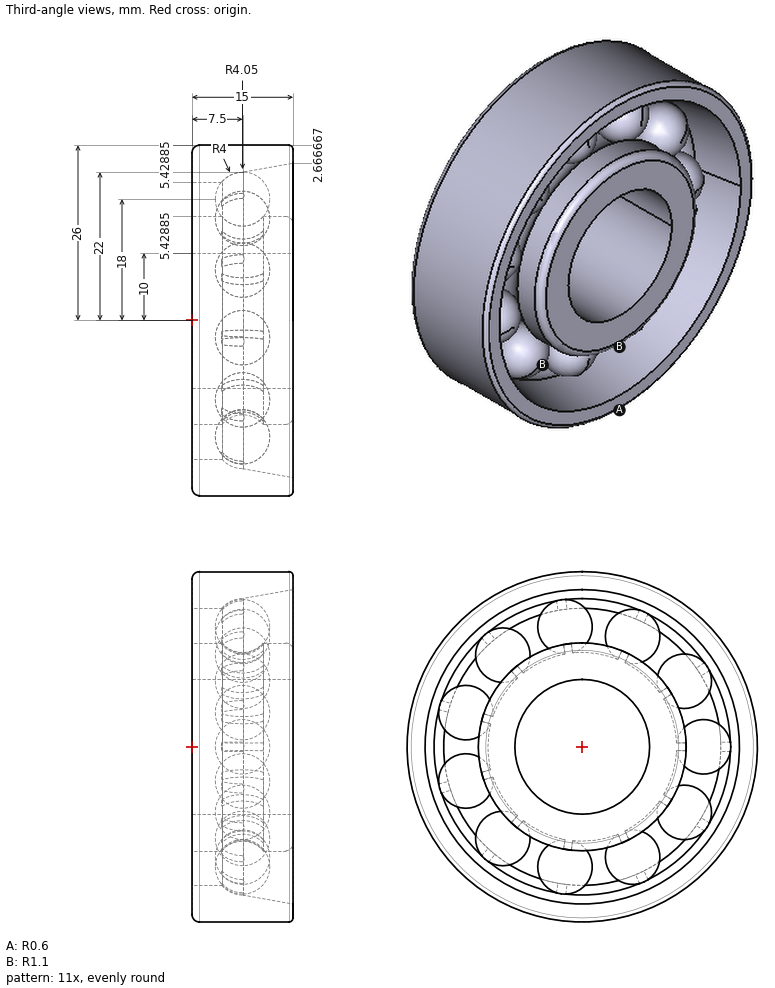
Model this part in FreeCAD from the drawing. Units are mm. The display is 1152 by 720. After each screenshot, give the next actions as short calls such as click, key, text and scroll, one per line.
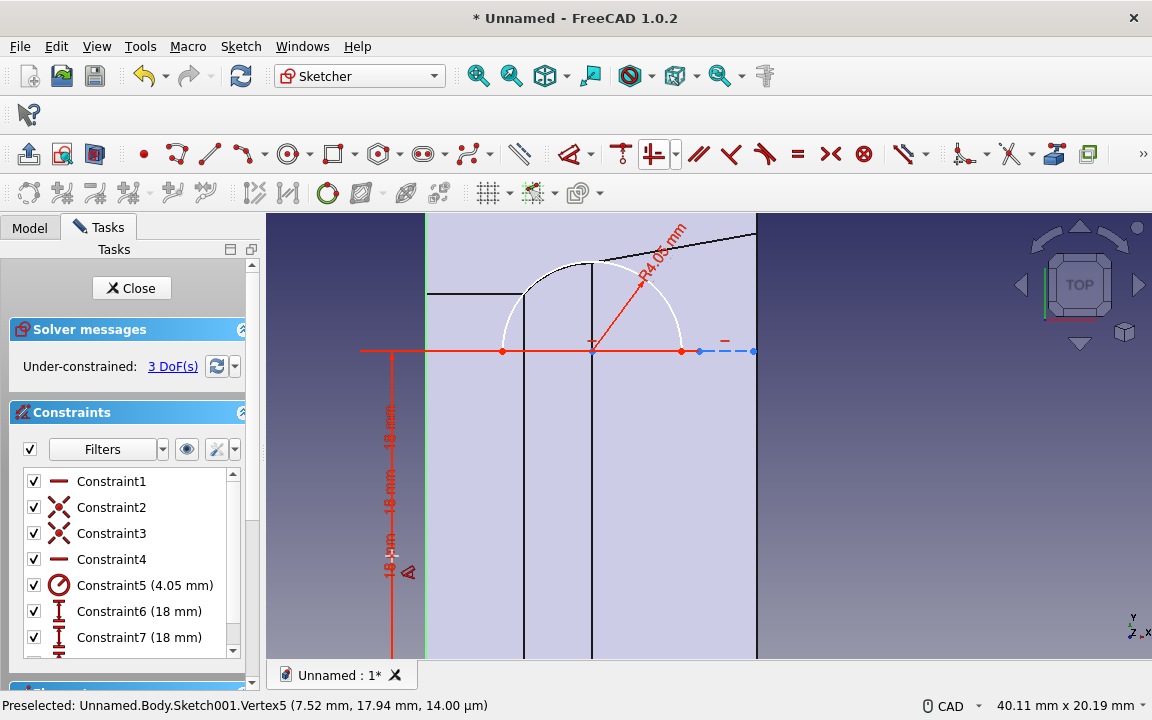
click(592, 351)
click(471, 317)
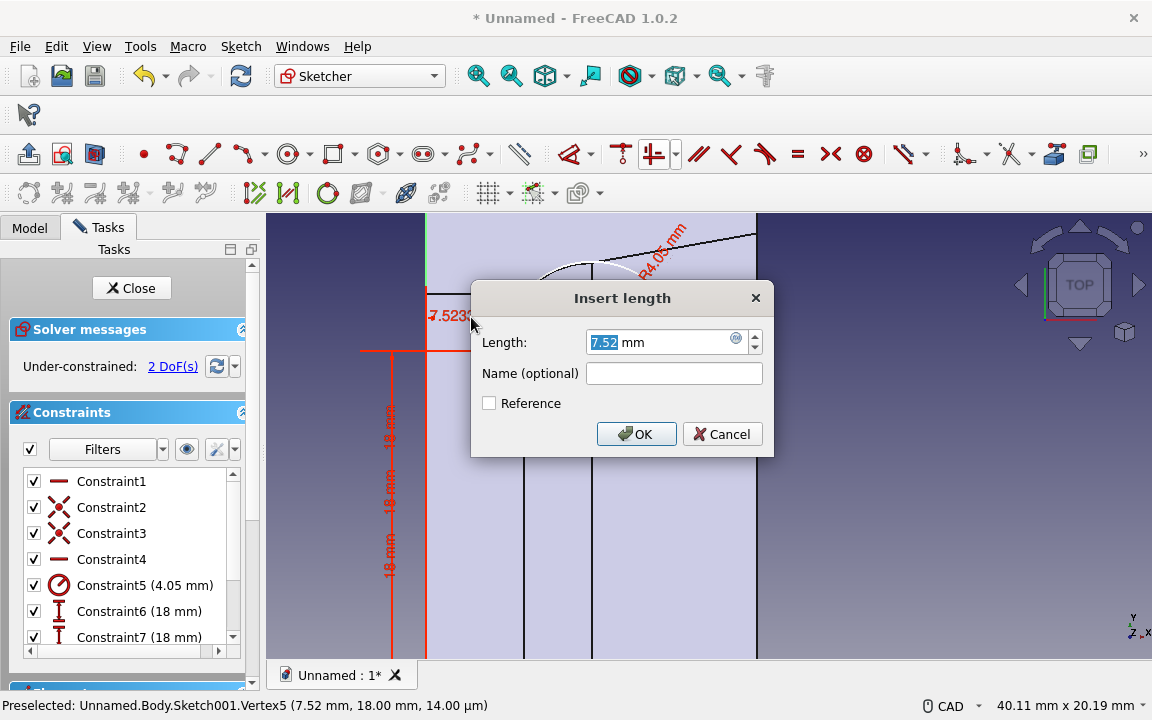
text(7.5)
key(Return)
key(Escape)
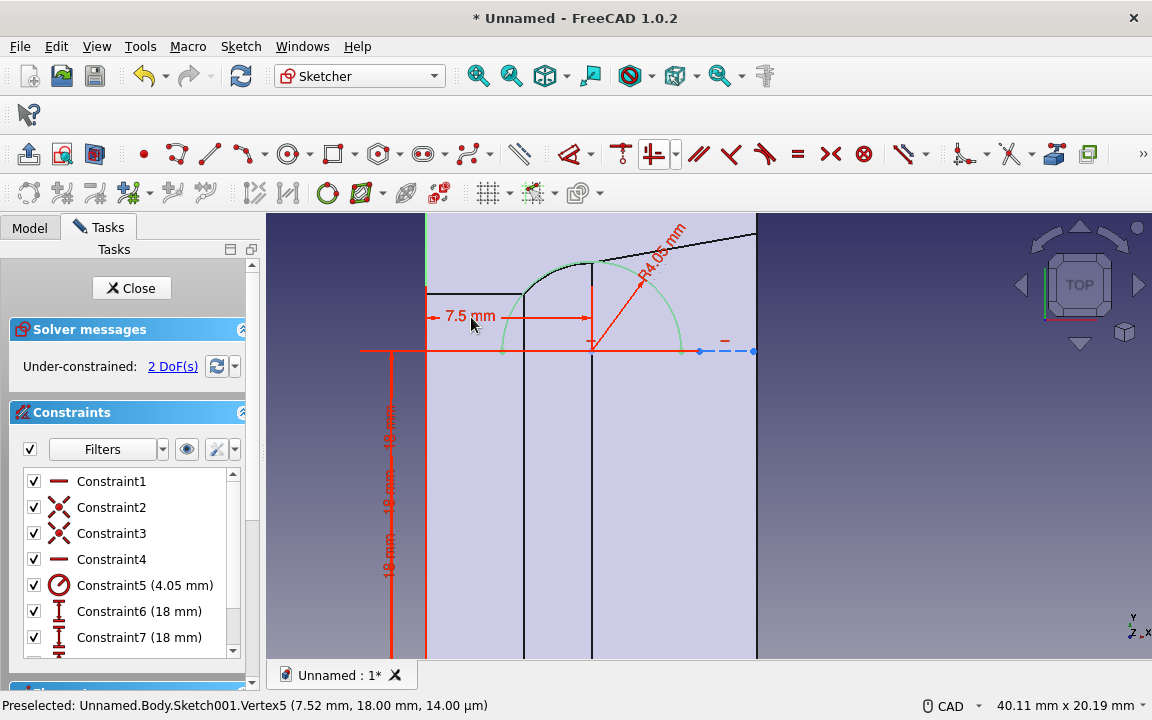
click(132, 288)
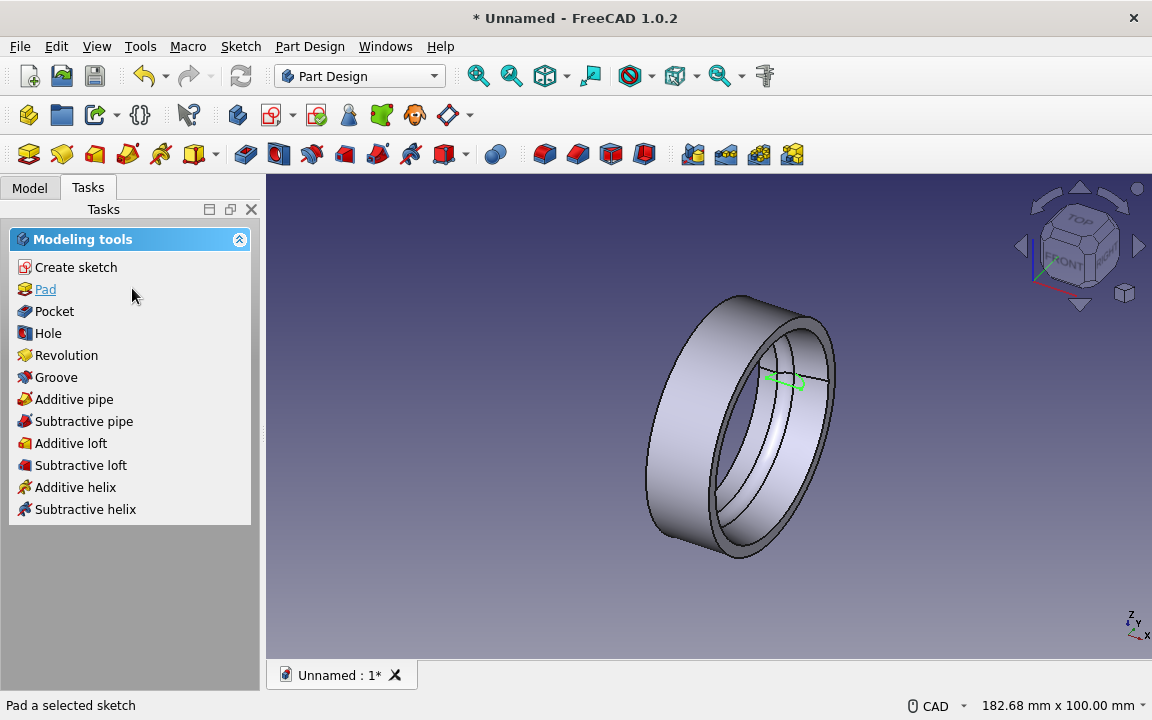
click(62, 154)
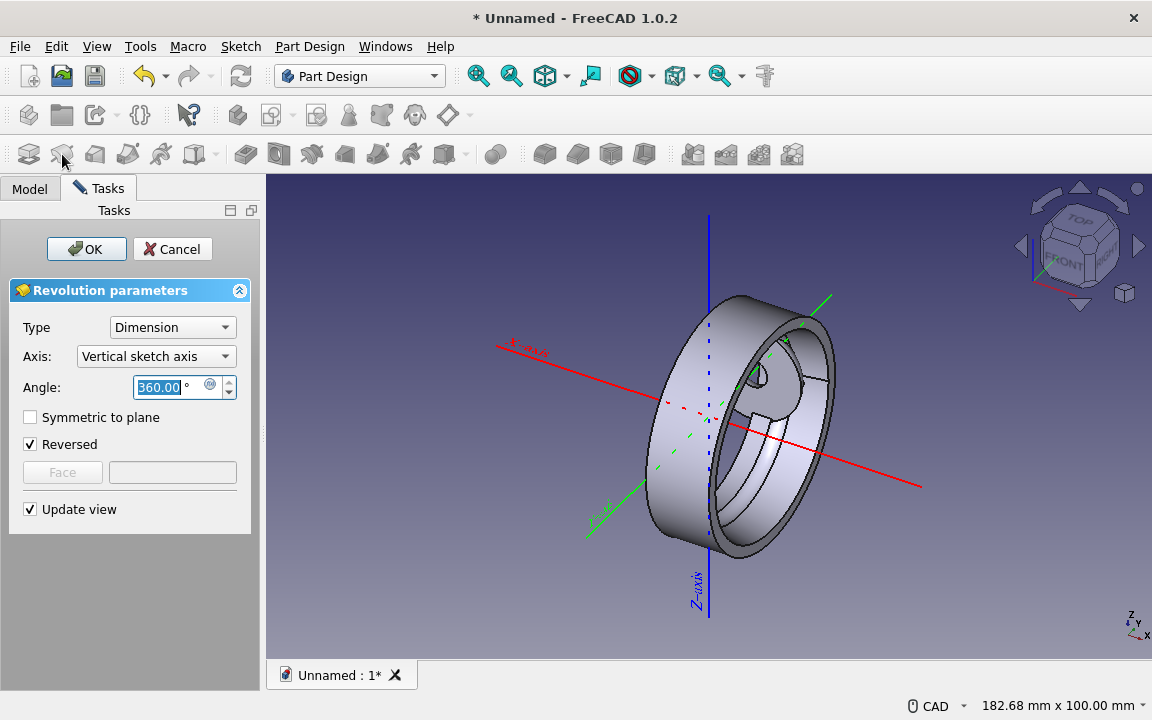
click(157, 356)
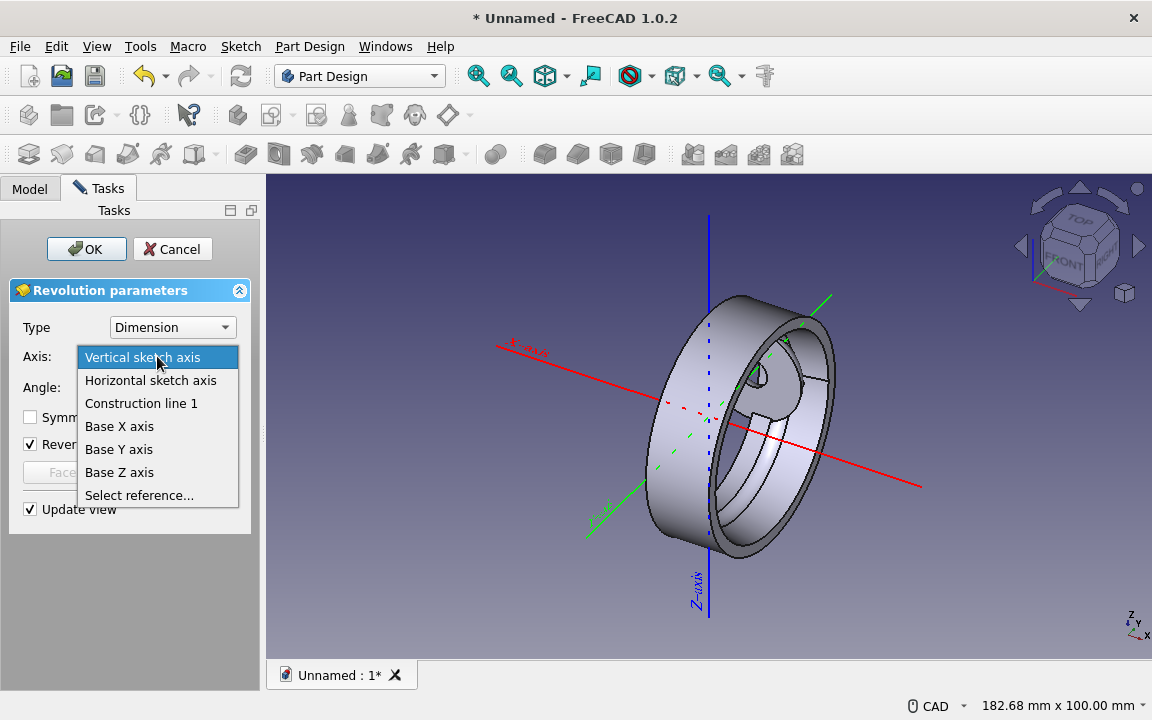
click(156, 404)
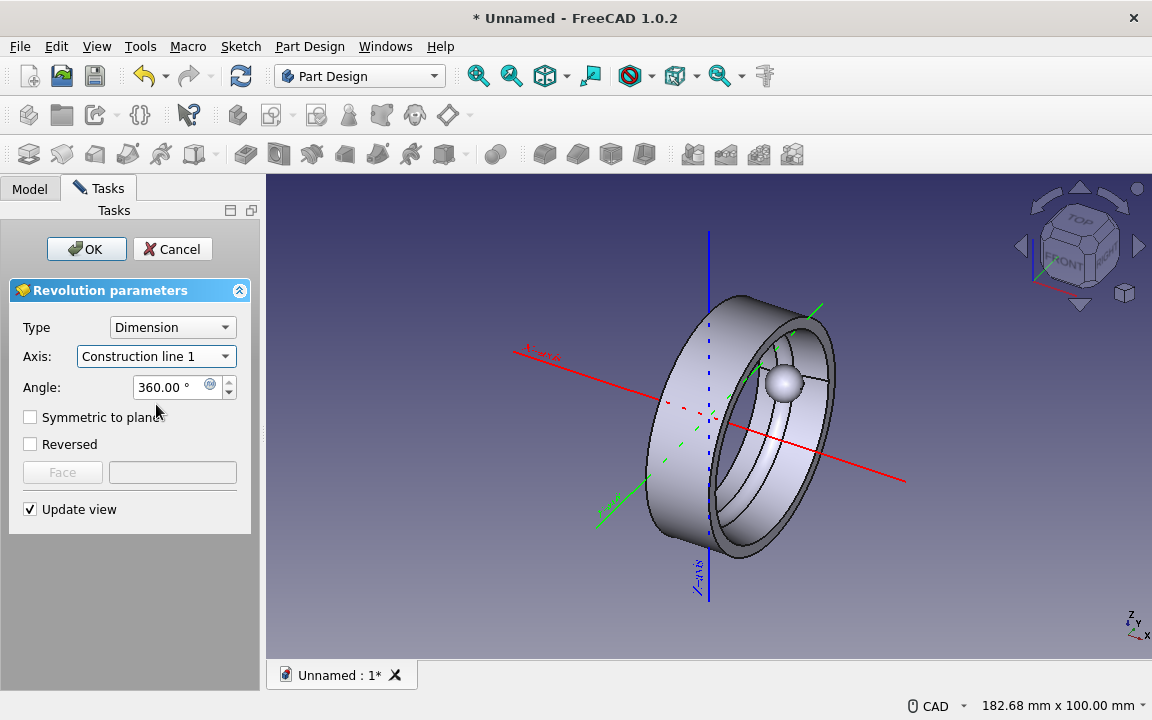
click(87, 249)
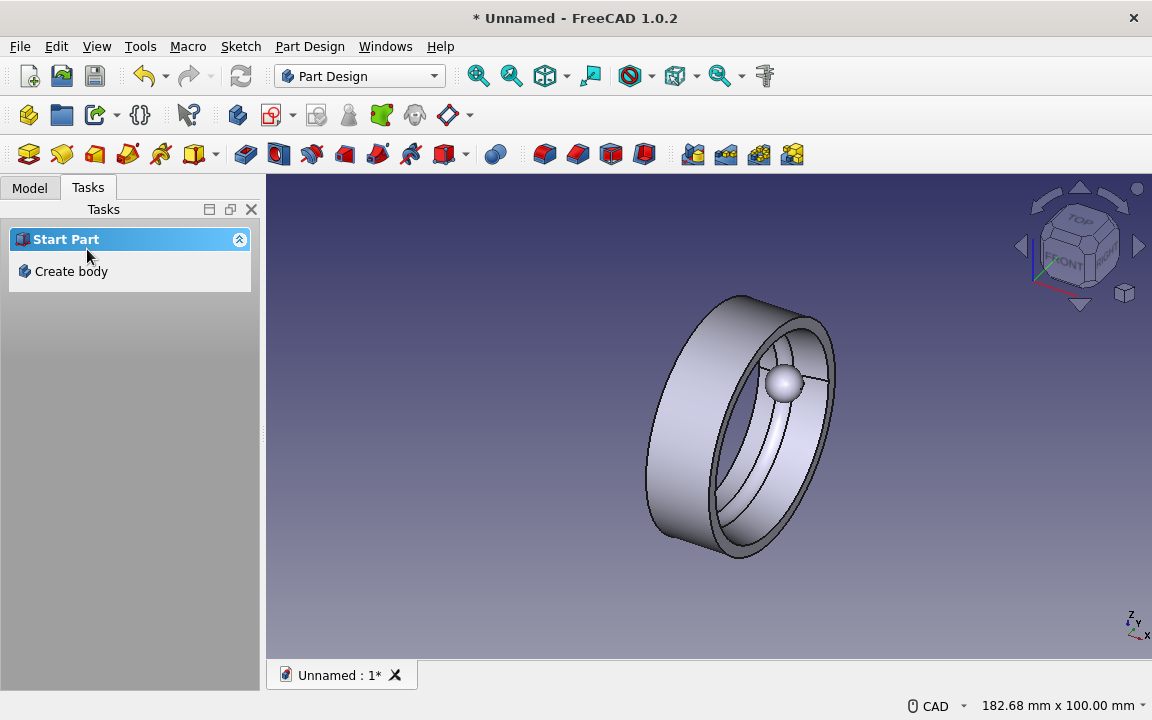
click(270, 116)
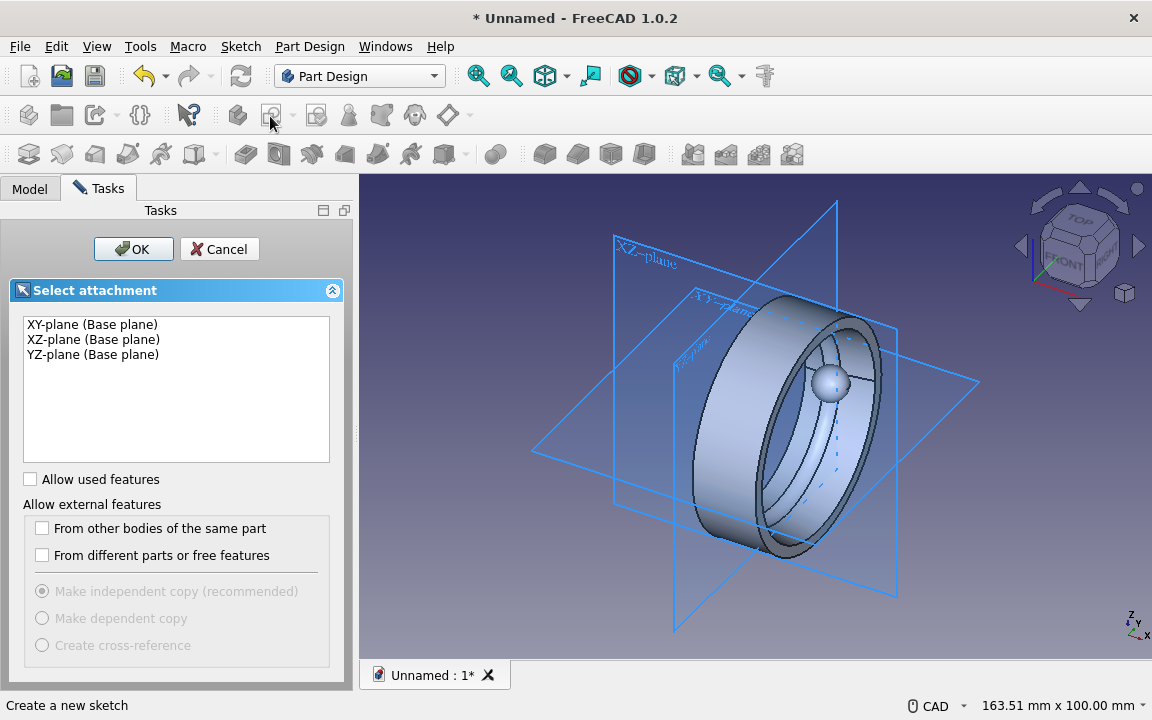
click(84, 324)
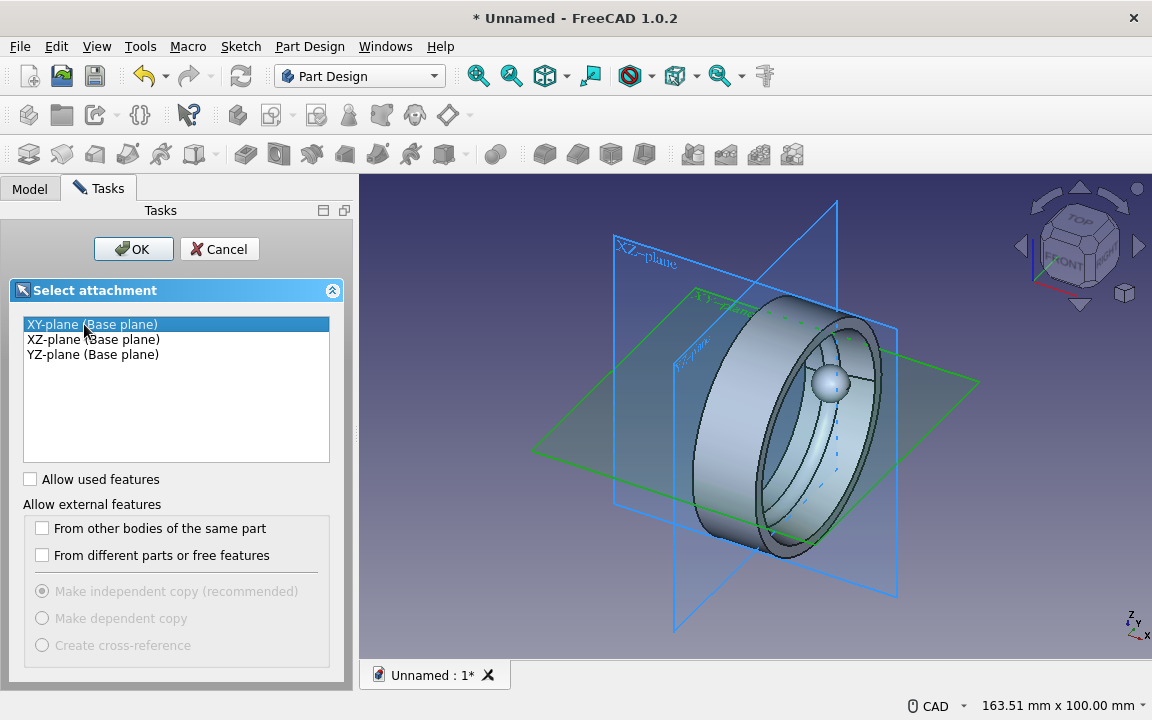
click(134, 249)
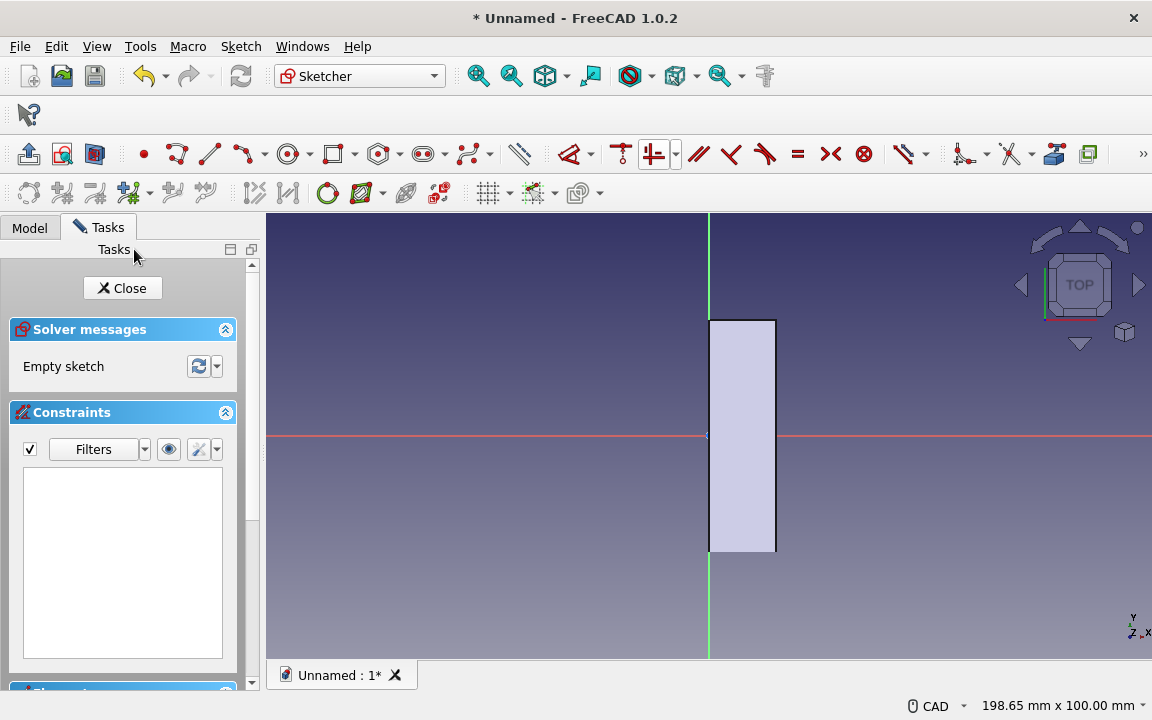
key(q)
key(s)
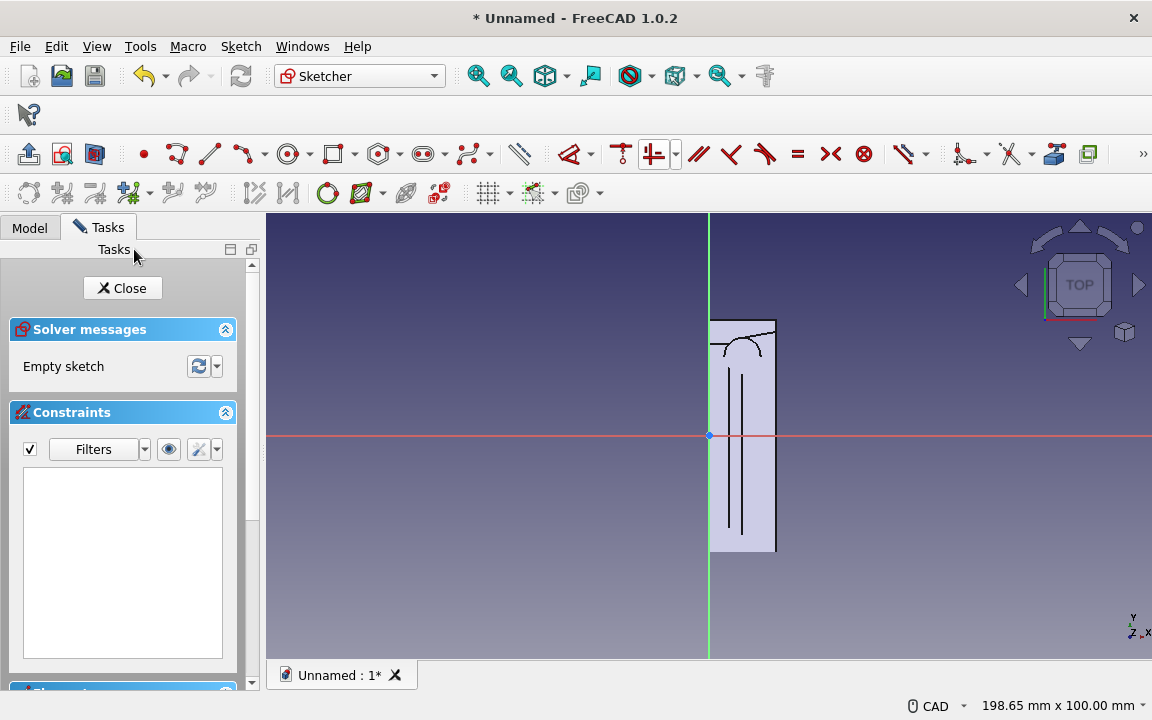
scroll(776, 390, up, 7)